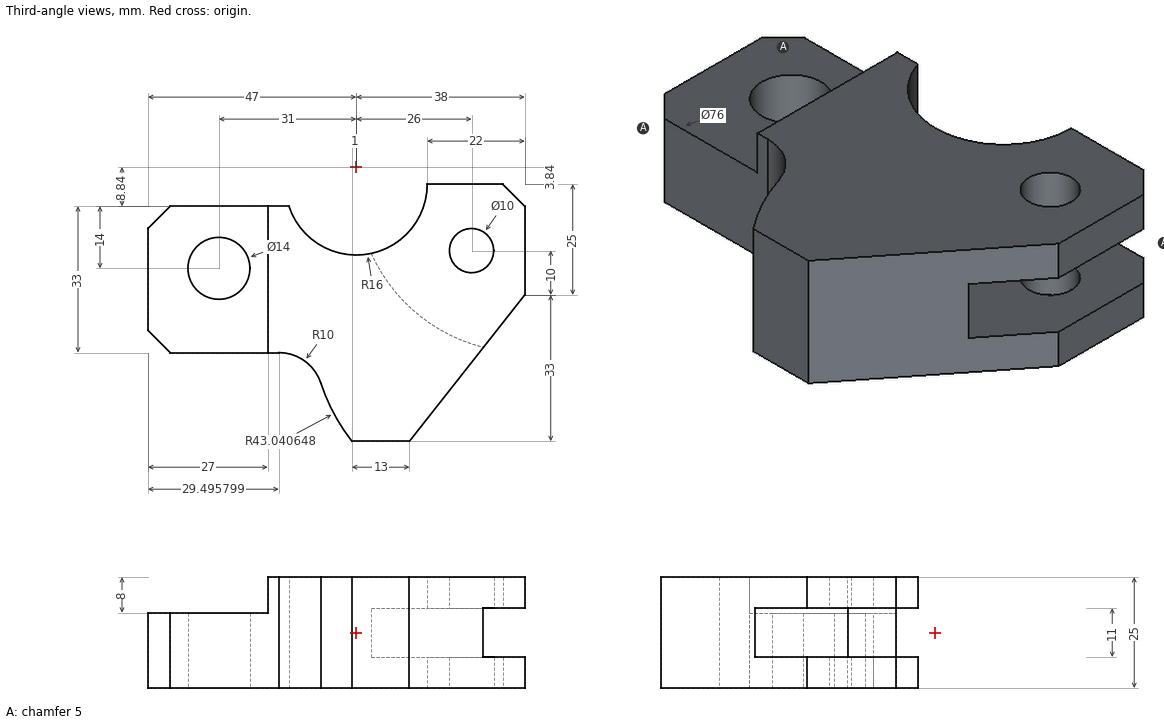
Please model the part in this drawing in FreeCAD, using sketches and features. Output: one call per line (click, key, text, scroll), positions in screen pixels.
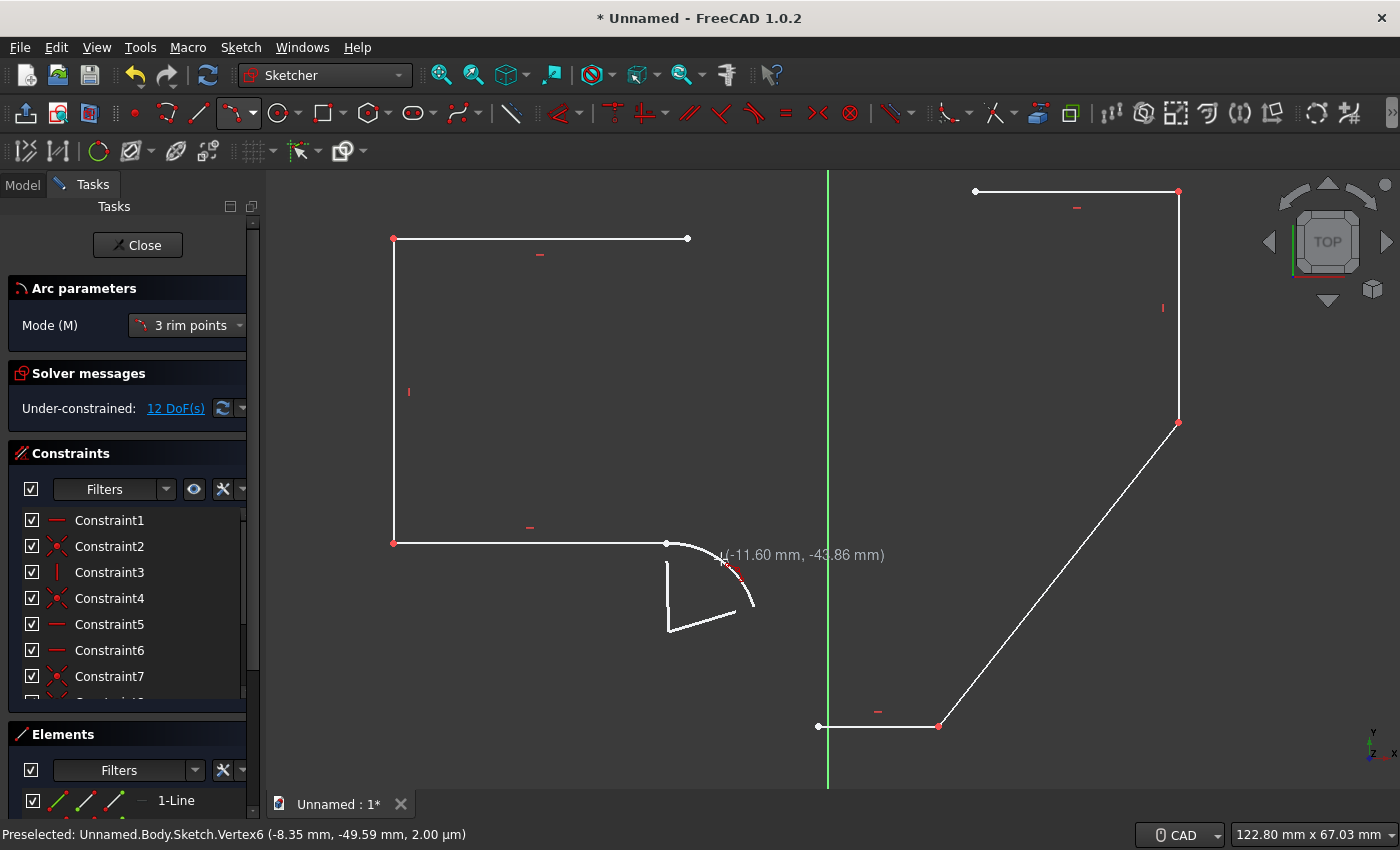
click(720, 559)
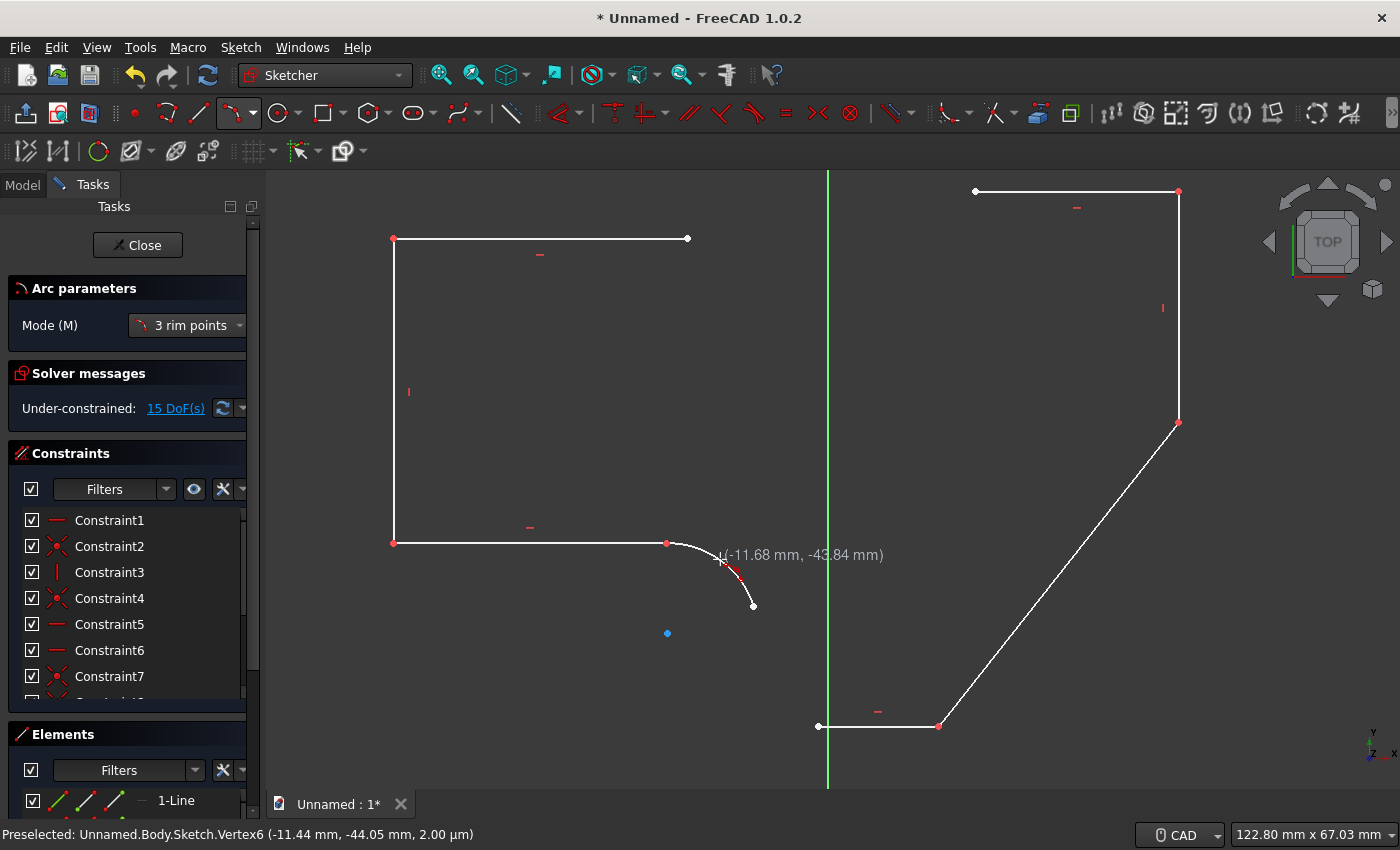
click(754, 606)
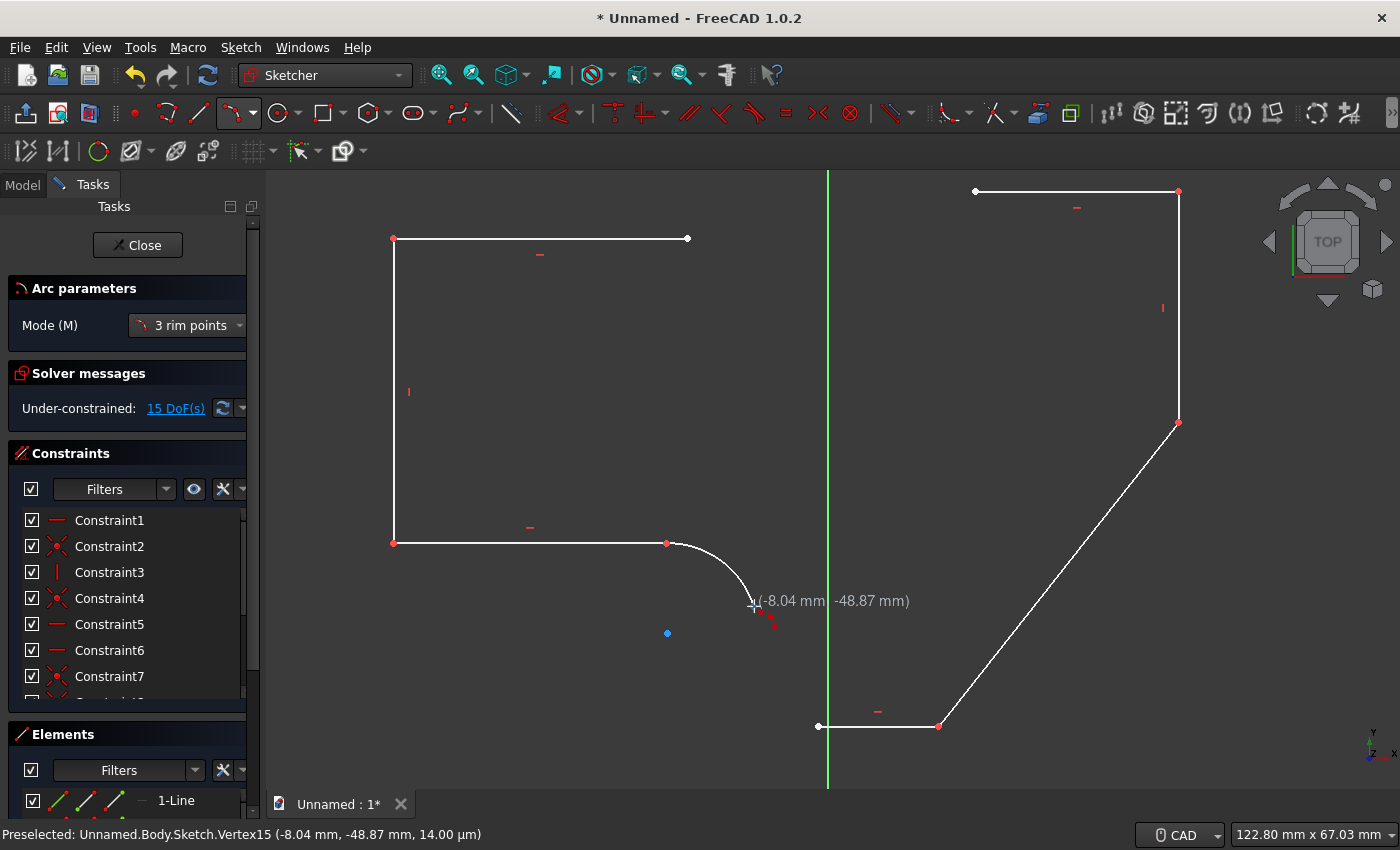
scroll(819, 726, up, 3)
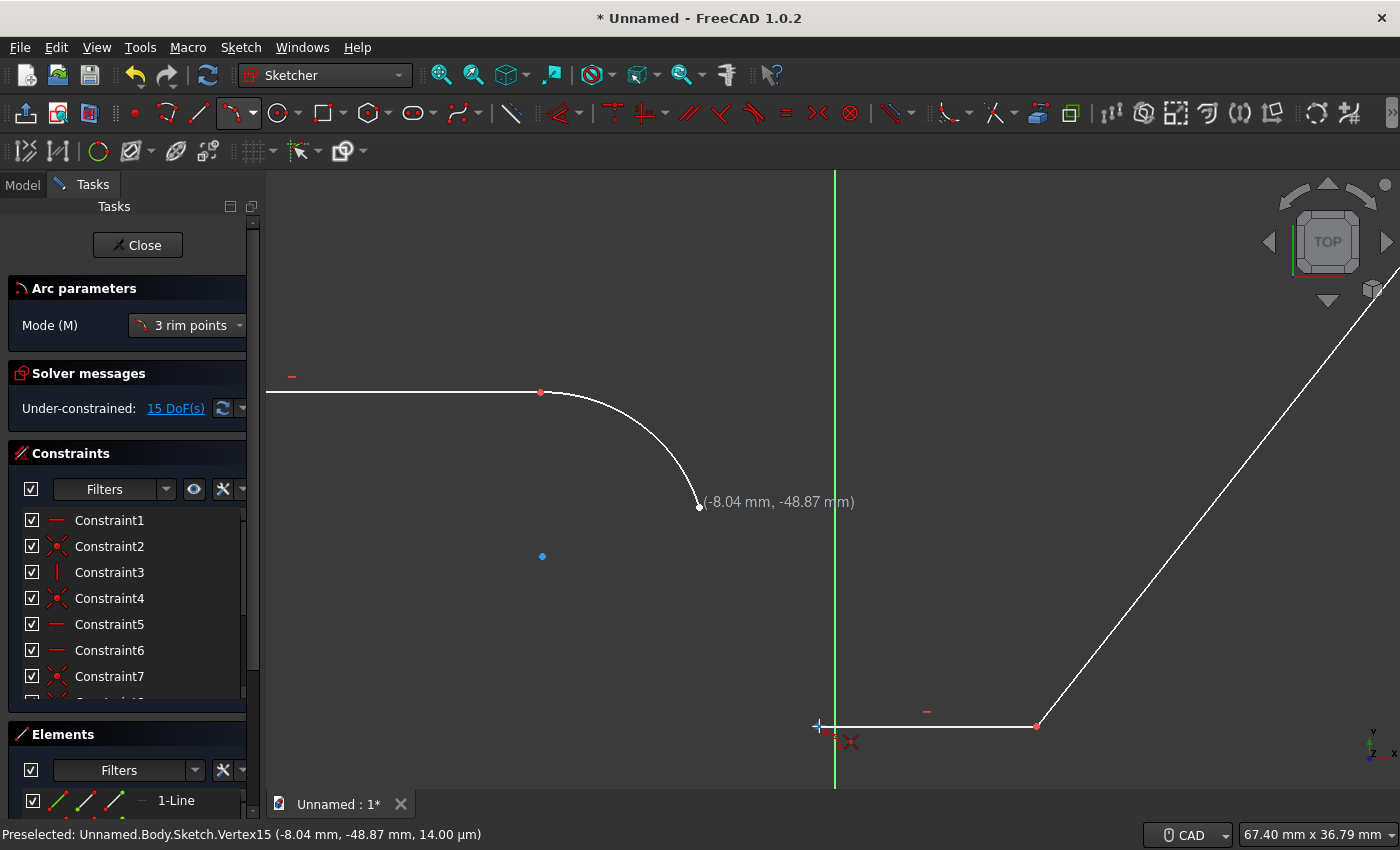
click(818, 727)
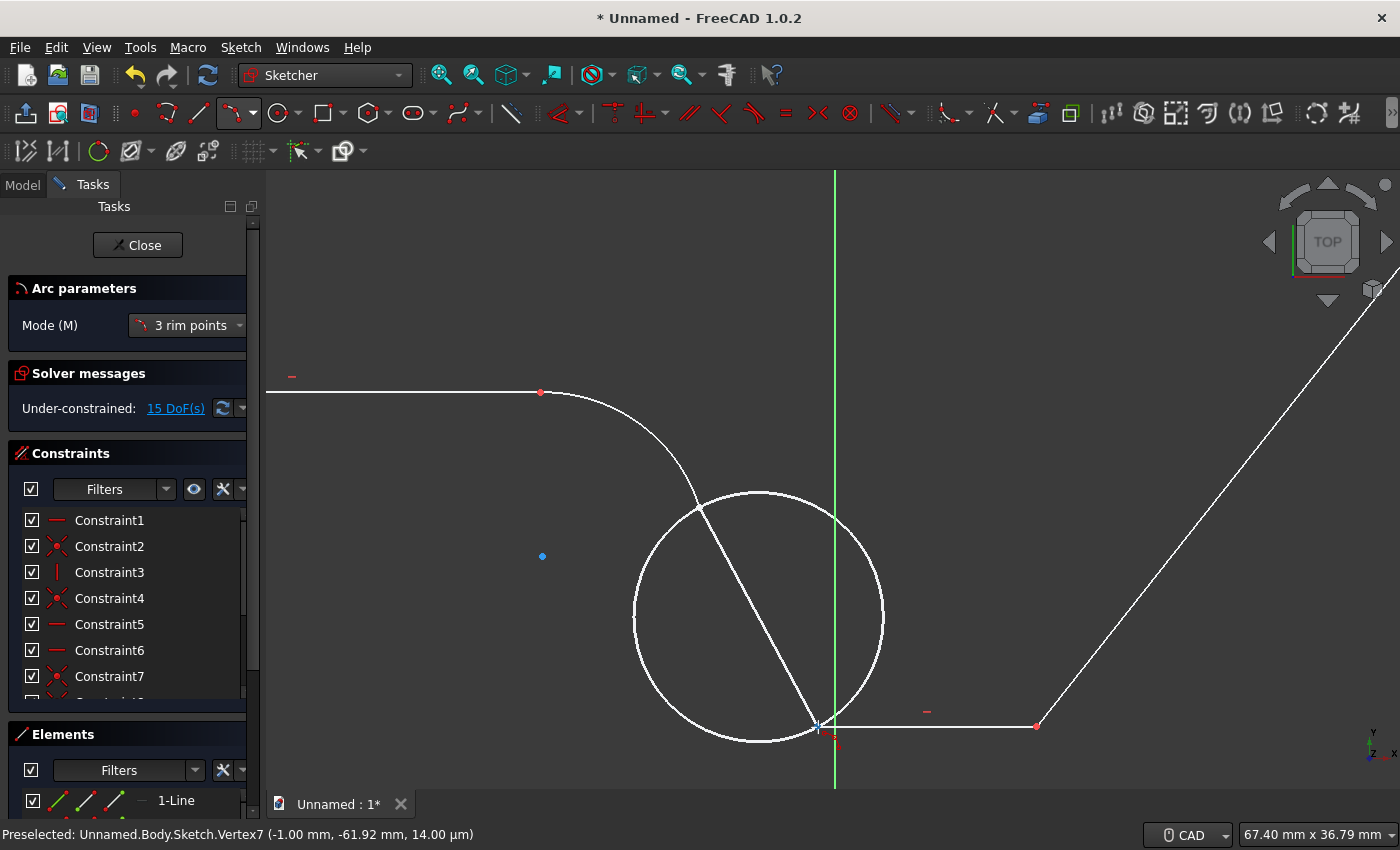
scroll(749, 620, up, 2)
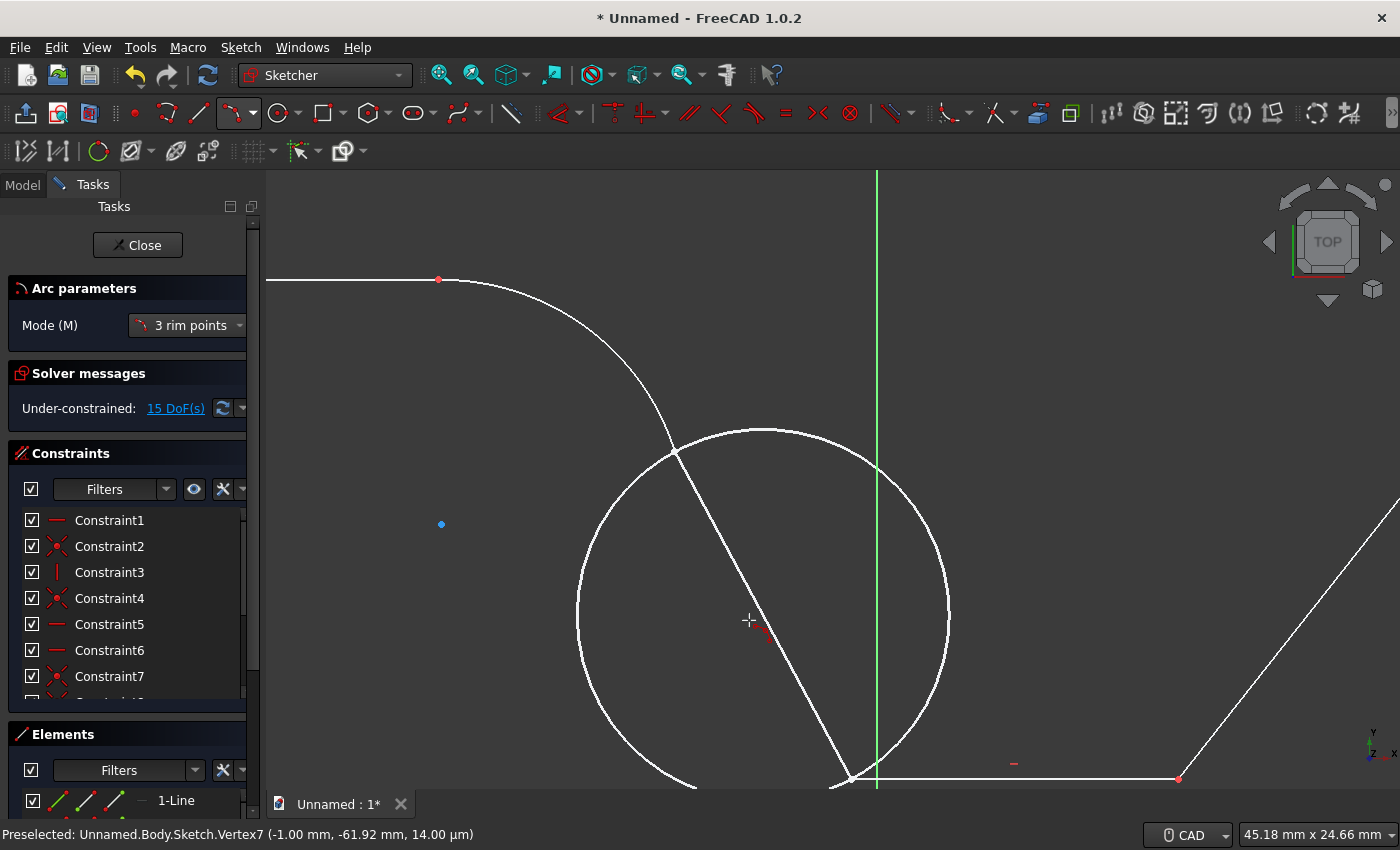
click(749, 620)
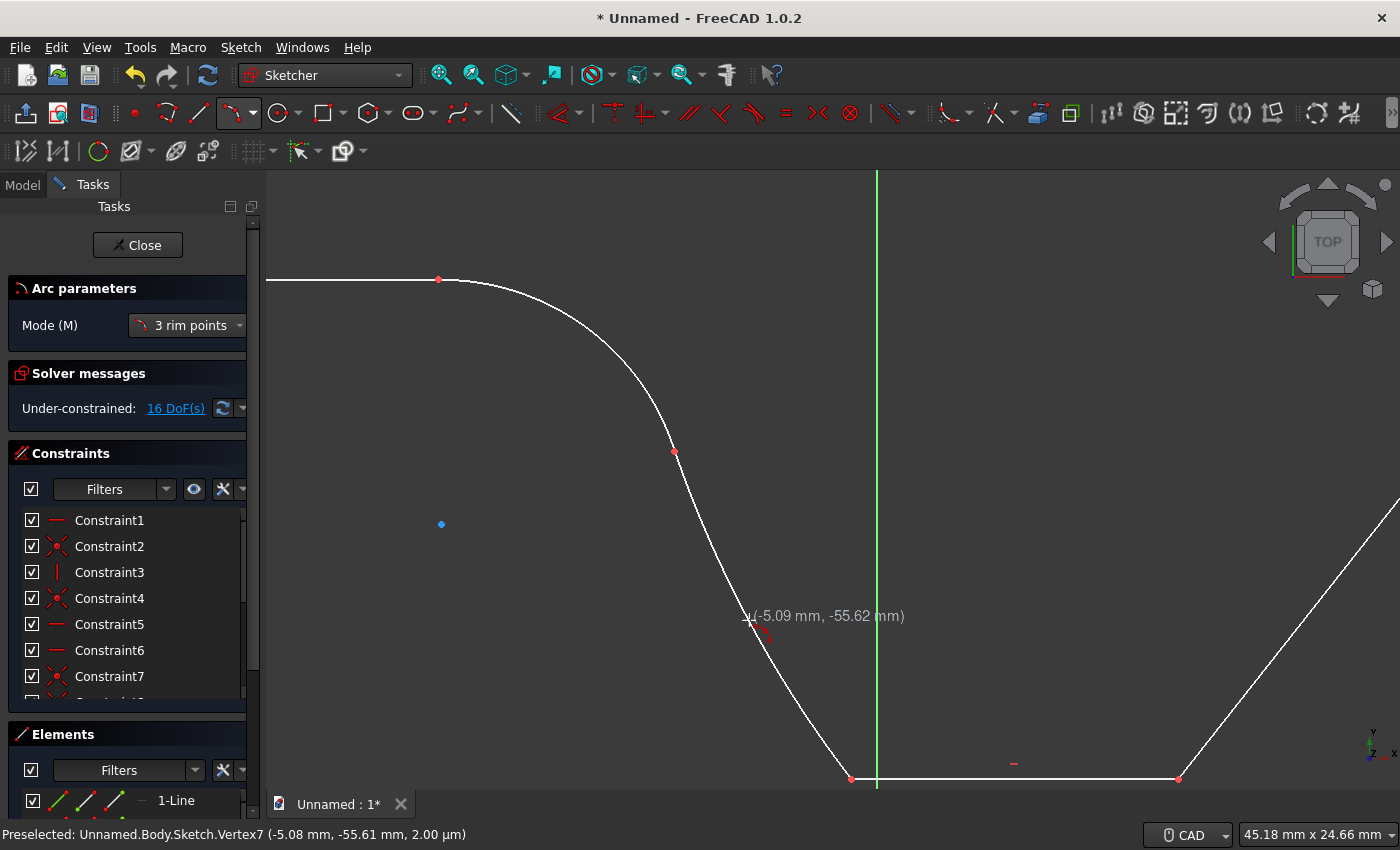
scroll(765, 636, down, 7)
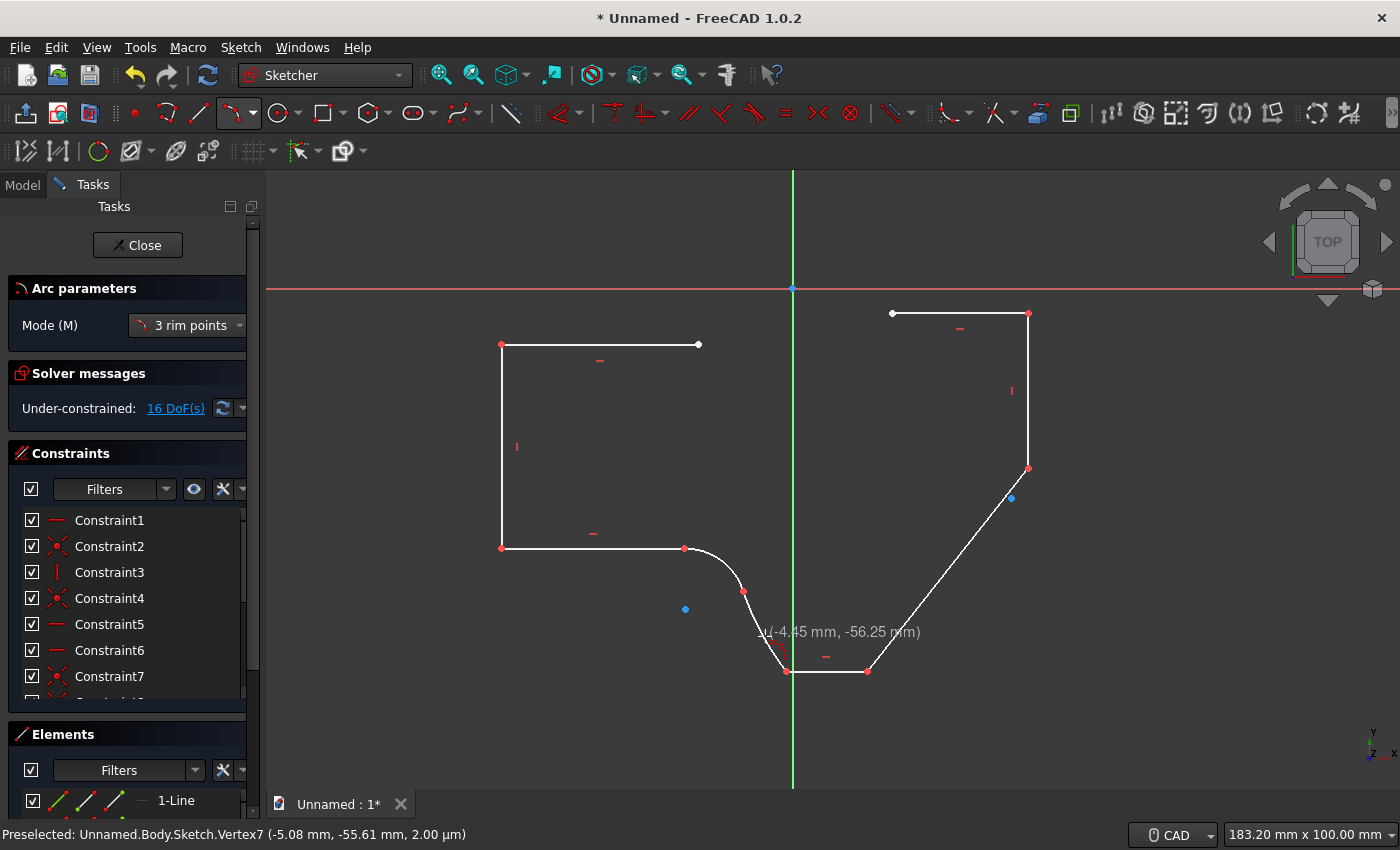
click(892, 313)
click(699, 345)
click(809, 410)